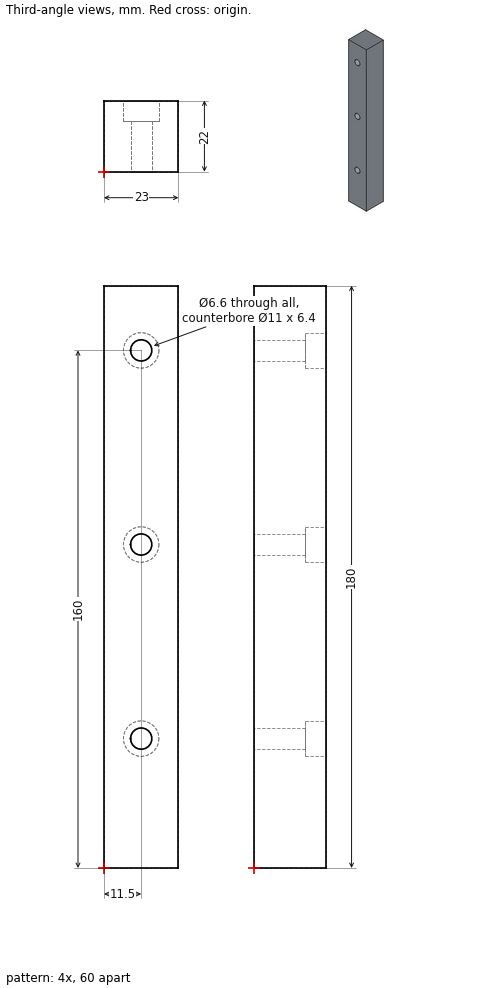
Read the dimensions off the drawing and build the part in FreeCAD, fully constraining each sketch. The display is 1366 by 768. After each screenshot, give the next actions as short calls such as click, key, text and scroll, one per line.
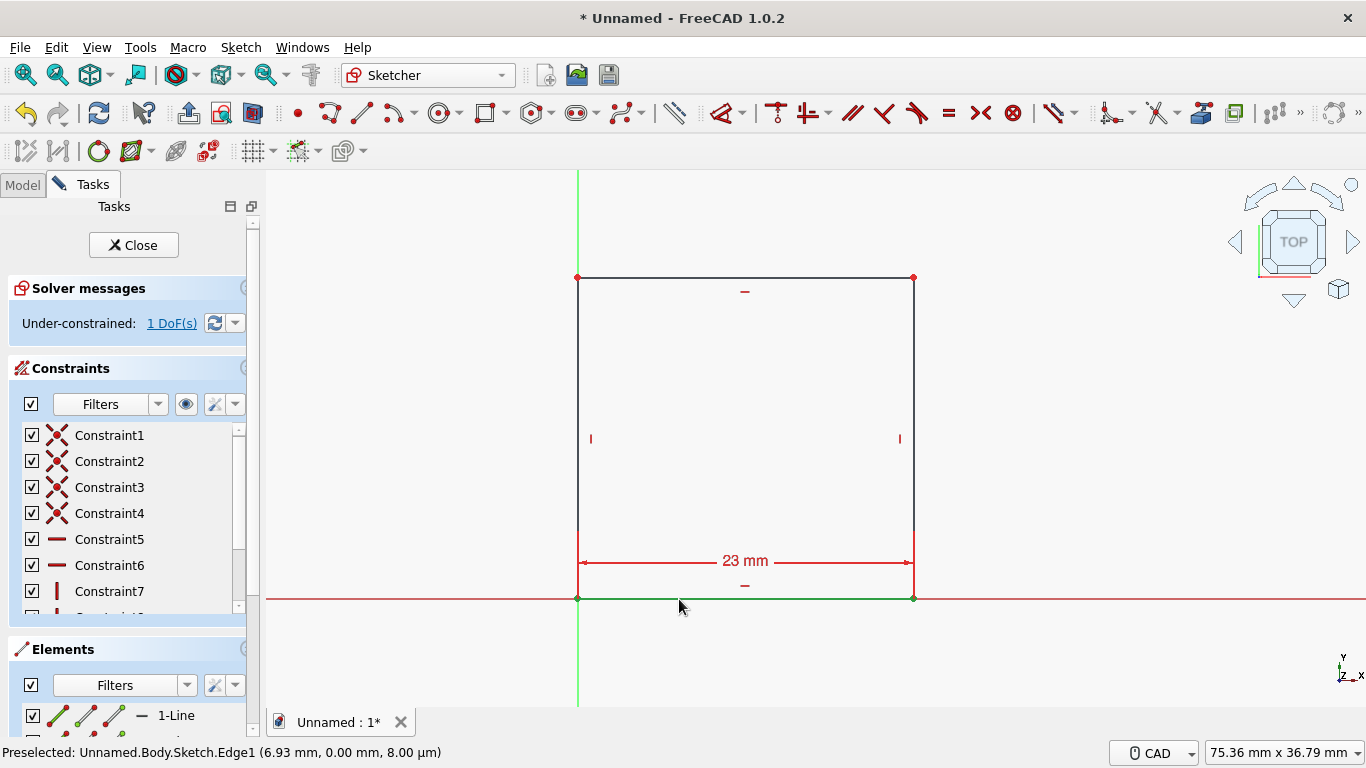
click(914, 502)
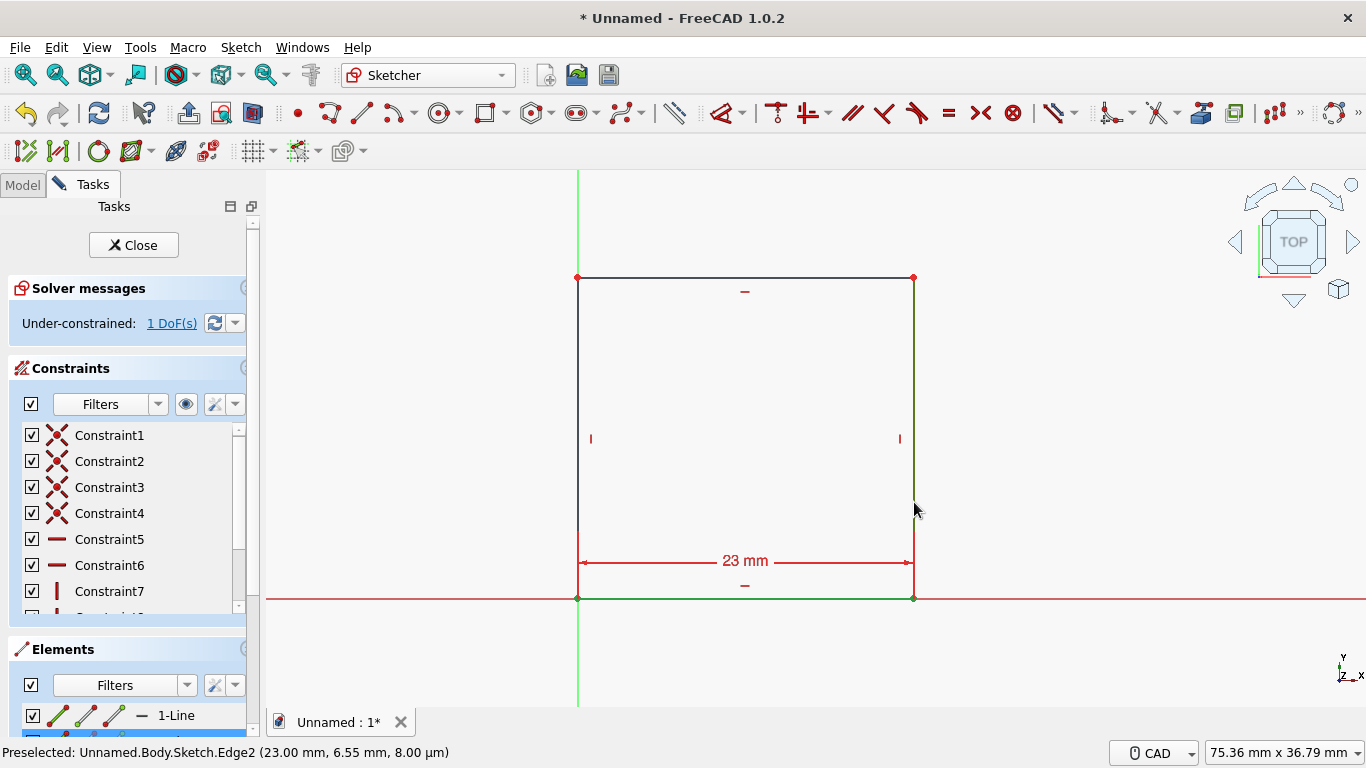
key(i)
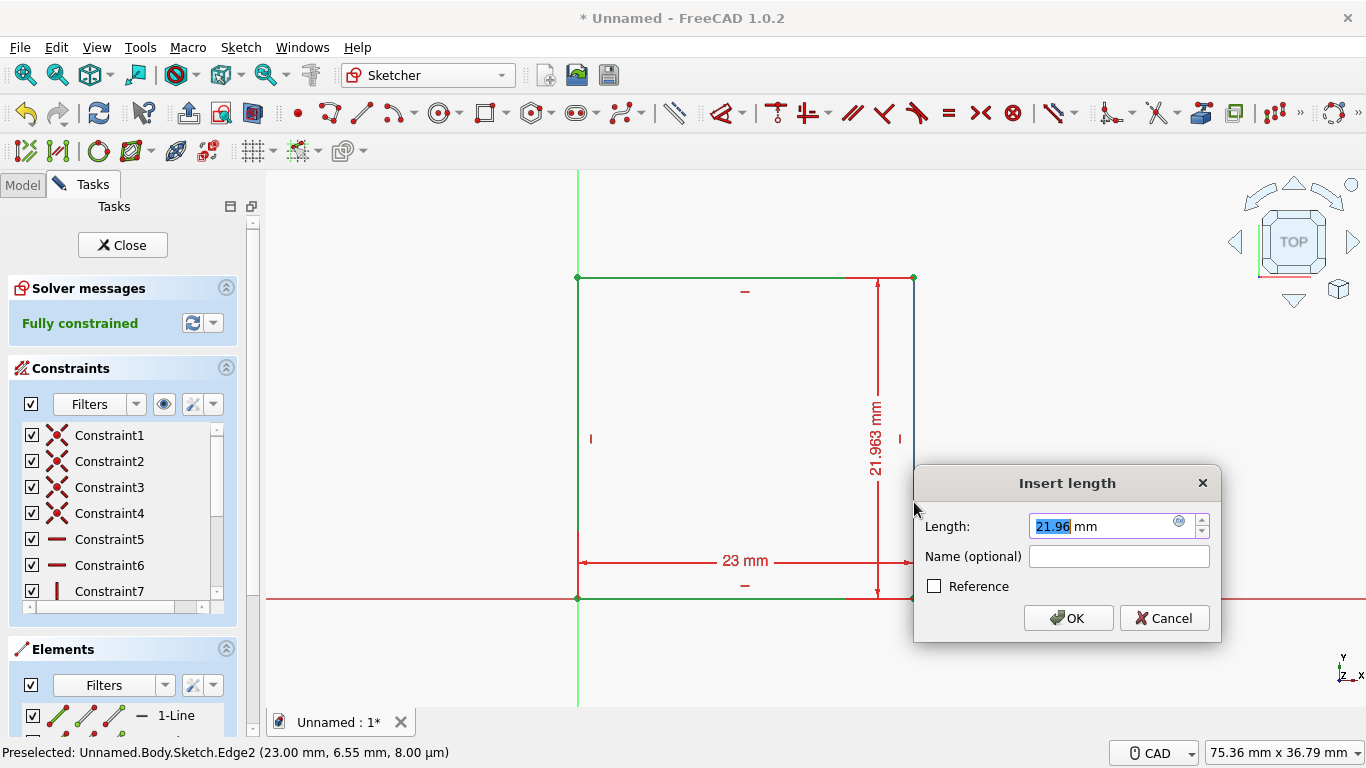
text(22)
key(Return)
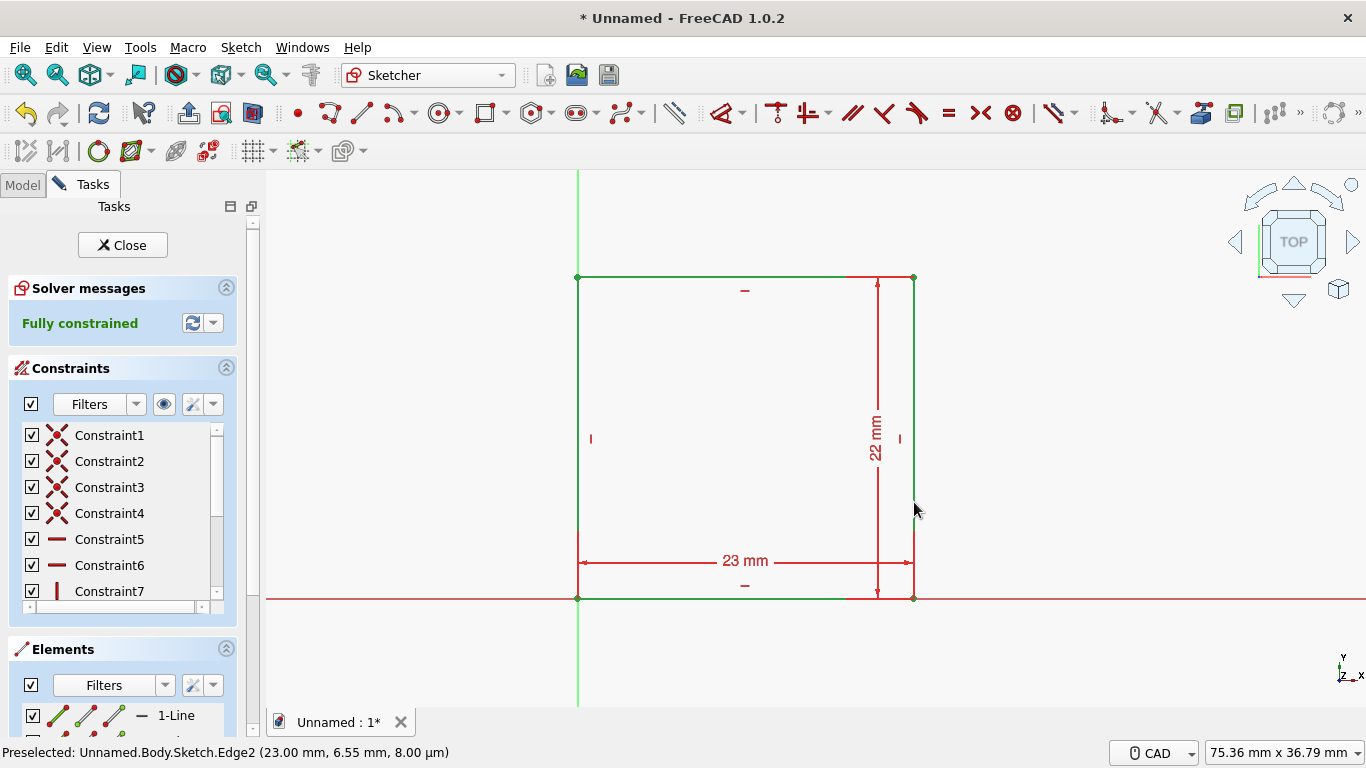
click(123, 245)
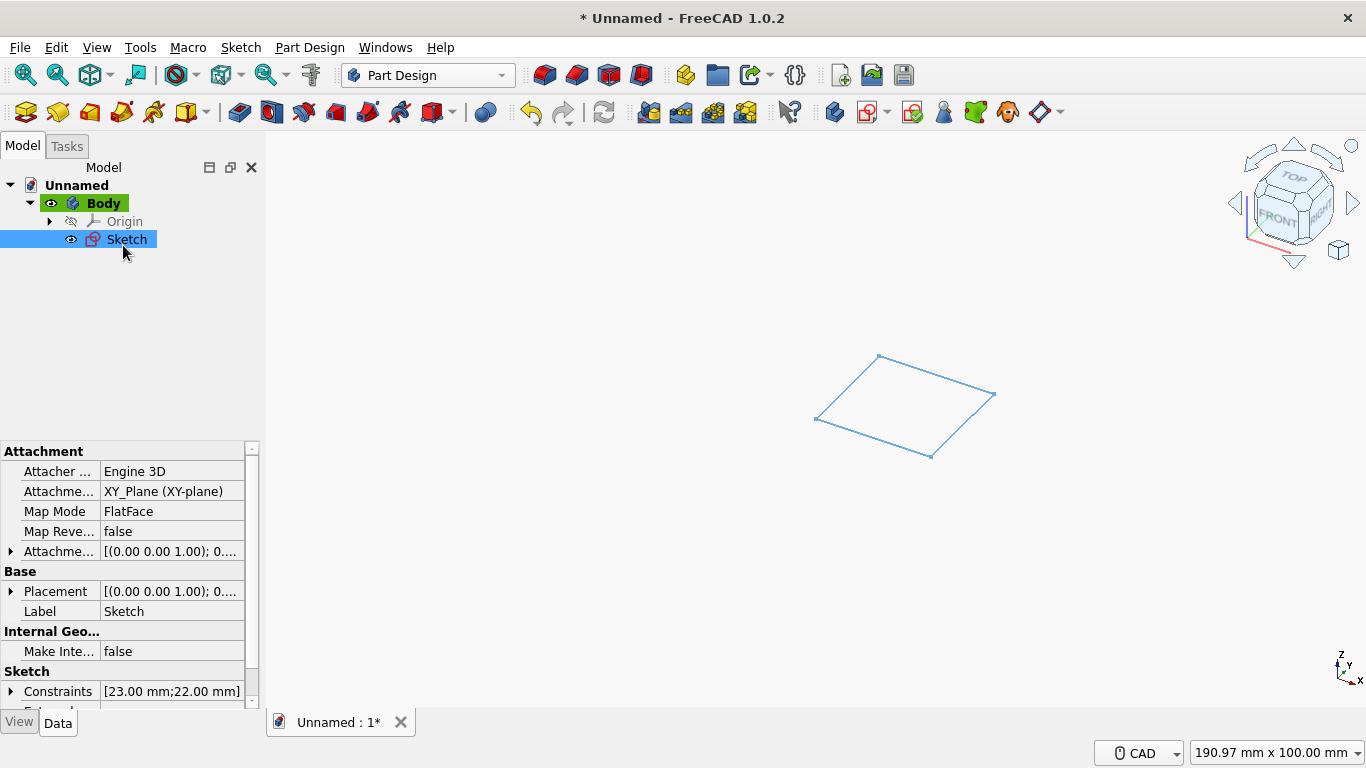
click(26, 112)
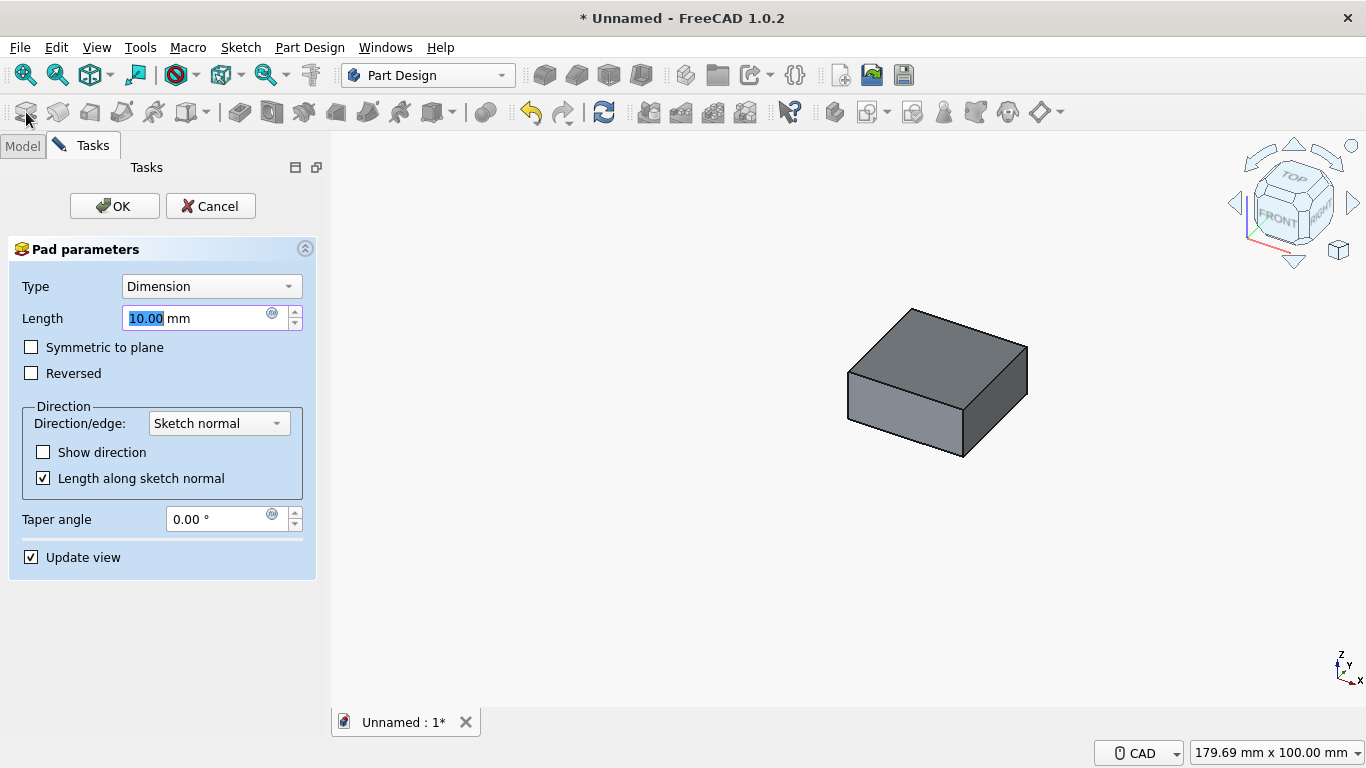
text(180)
key(Tab)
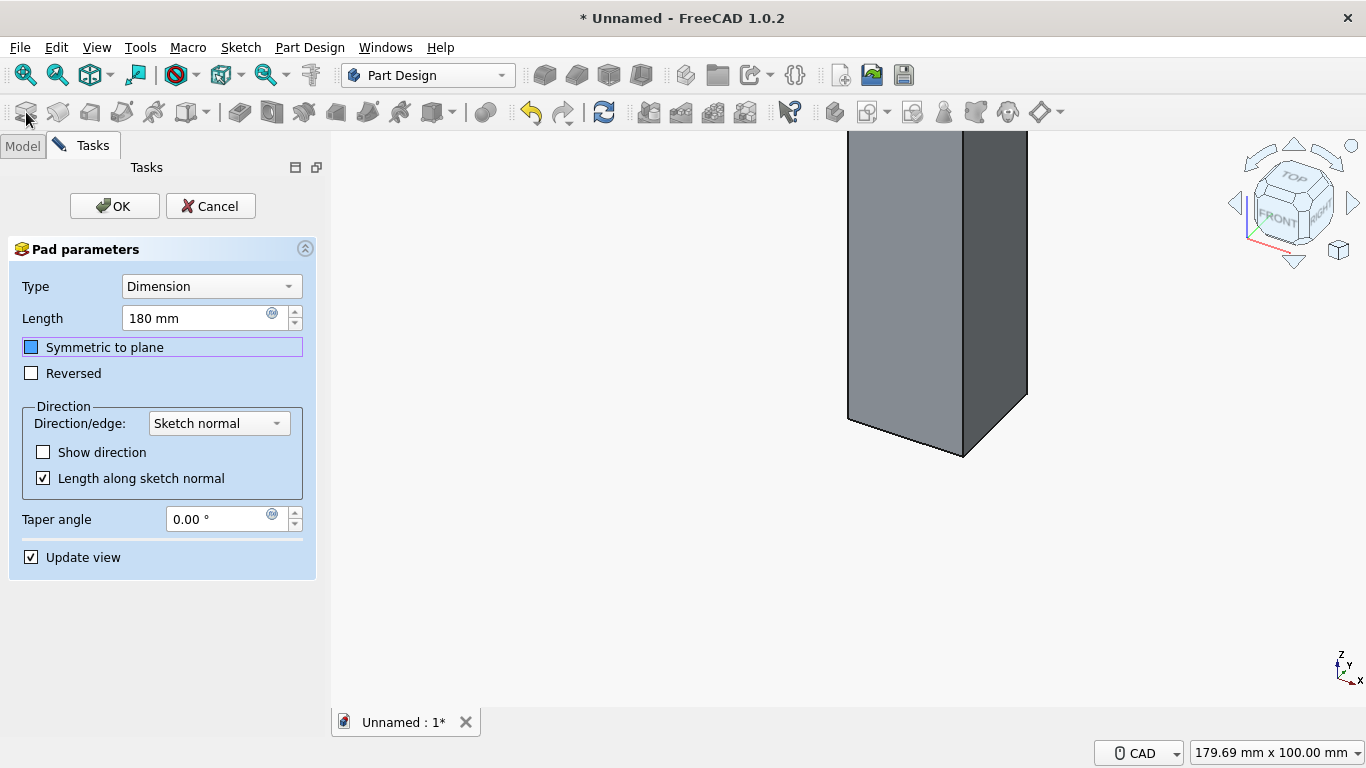
click(115, 206)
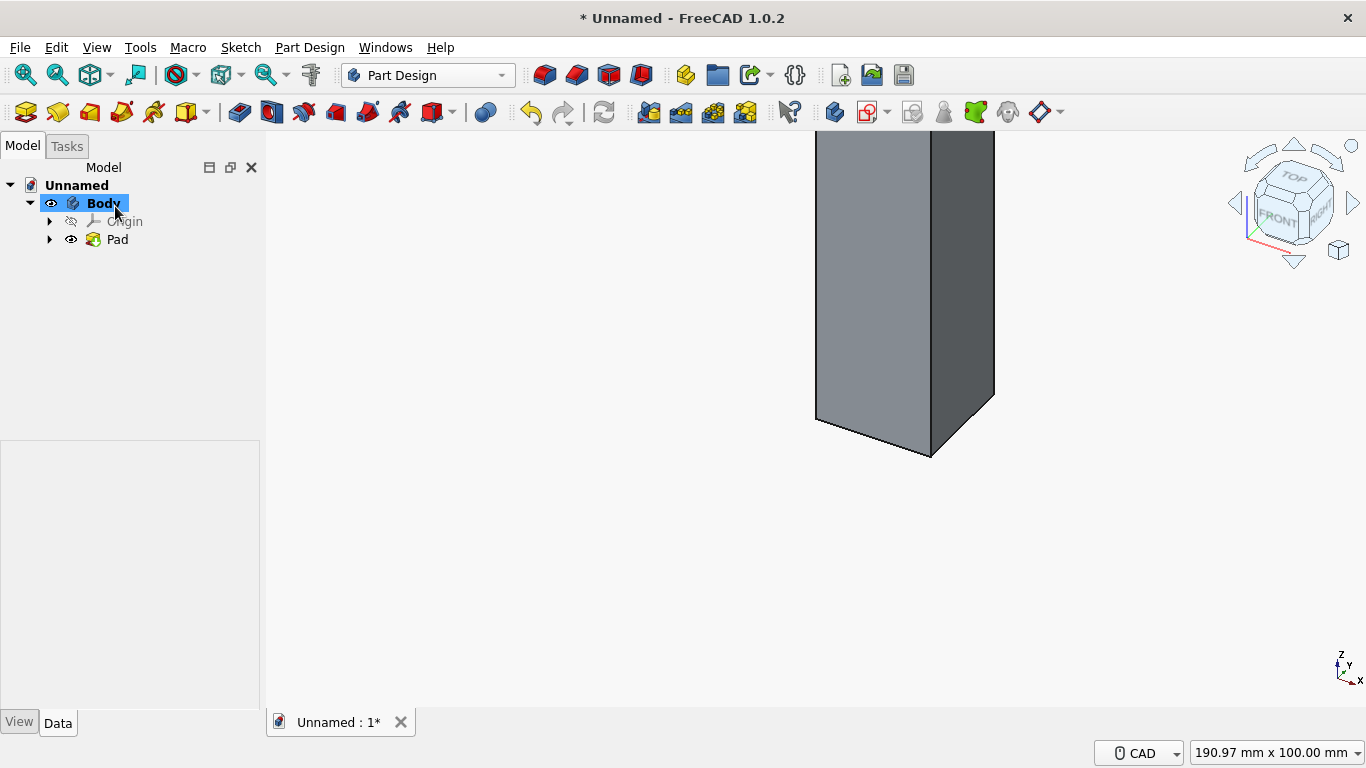
click(26, 76)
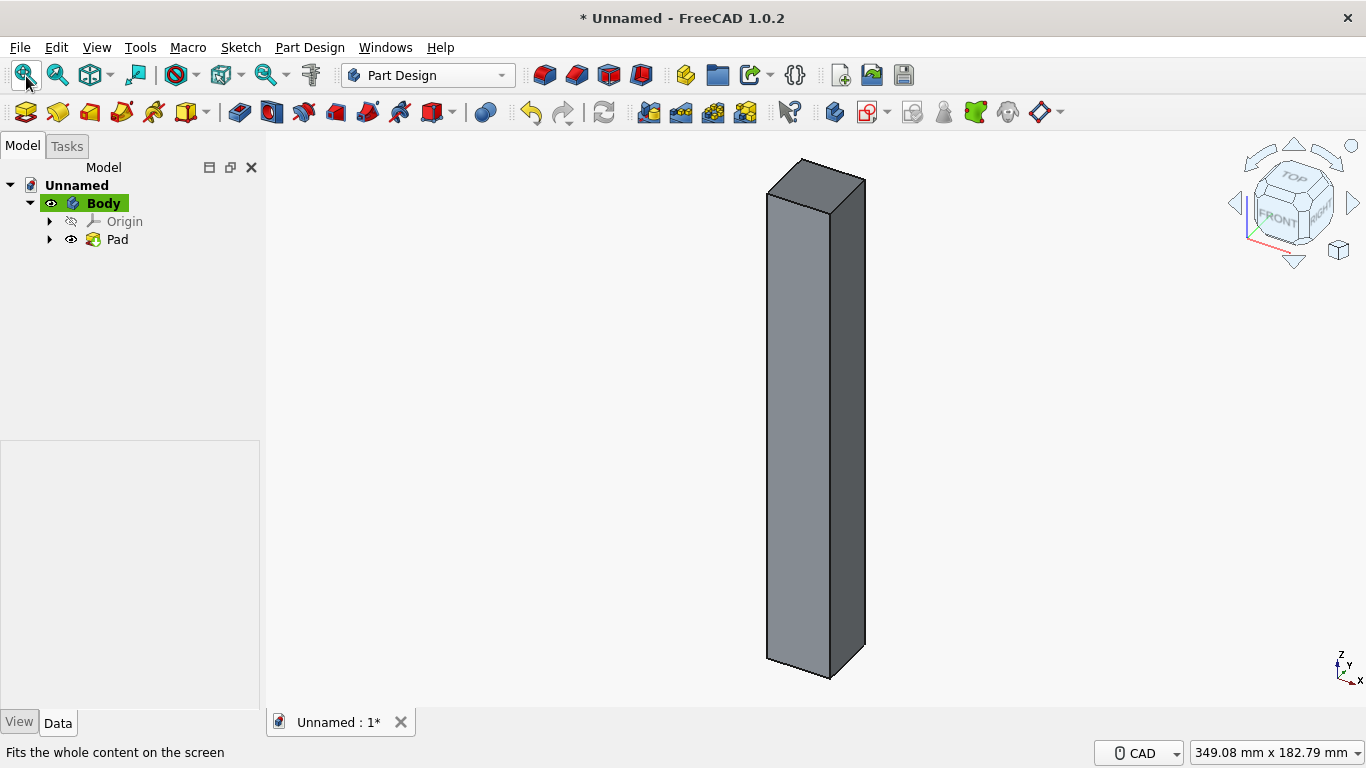
key(4)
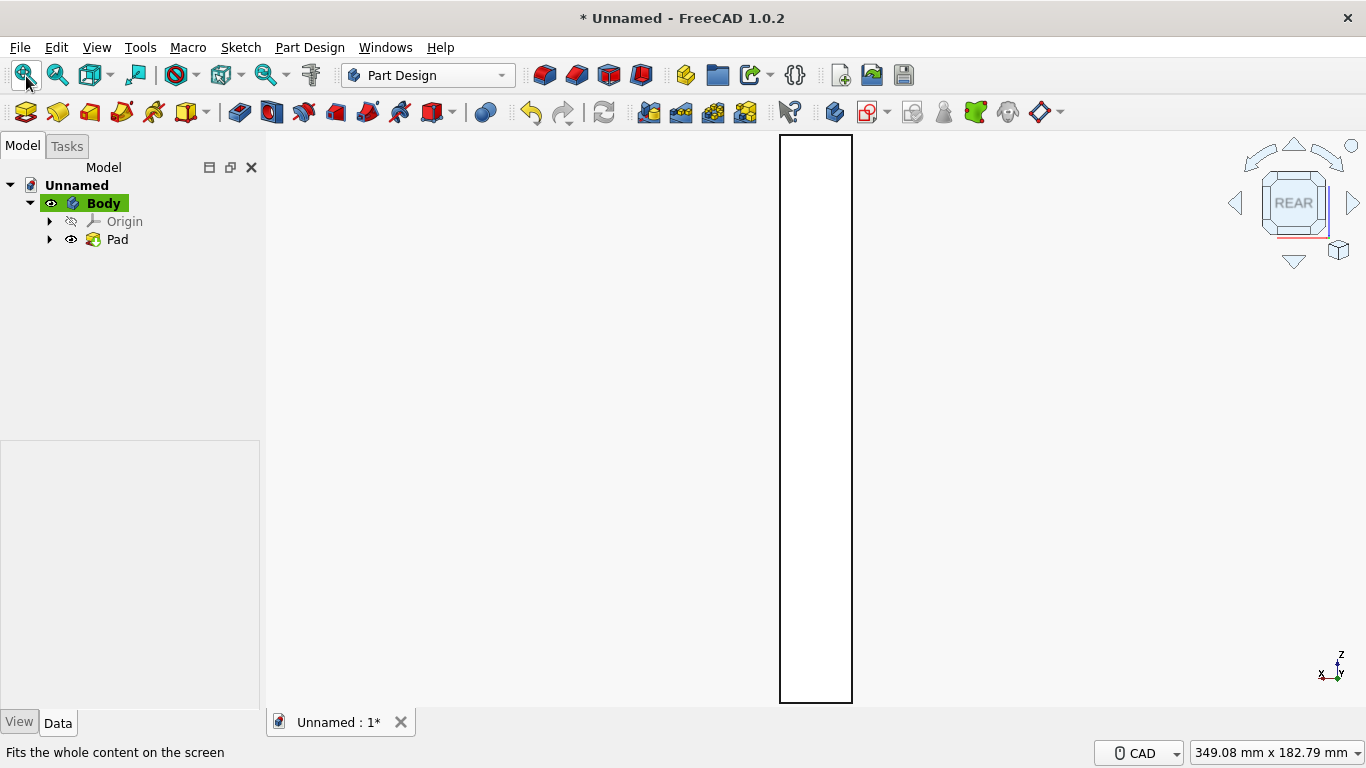
click(816, 175)